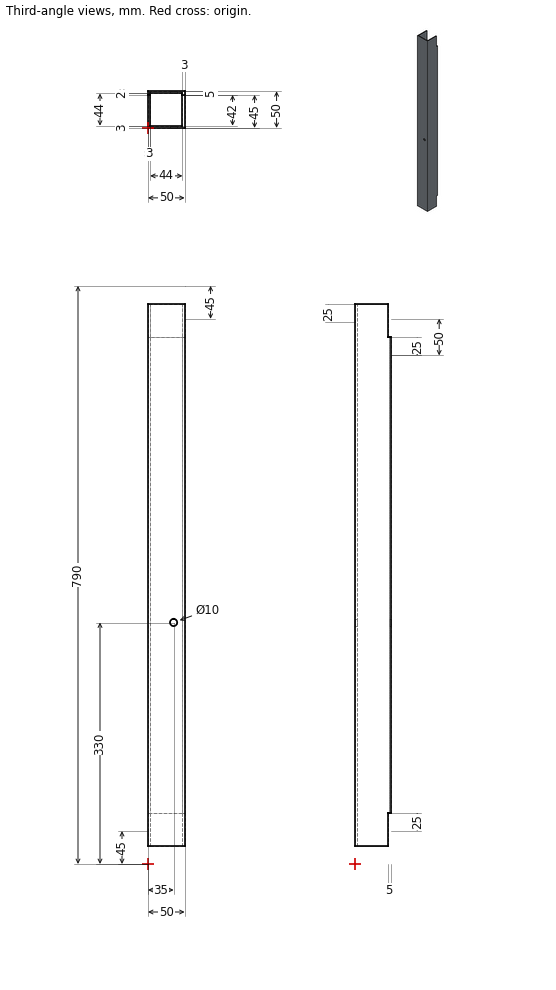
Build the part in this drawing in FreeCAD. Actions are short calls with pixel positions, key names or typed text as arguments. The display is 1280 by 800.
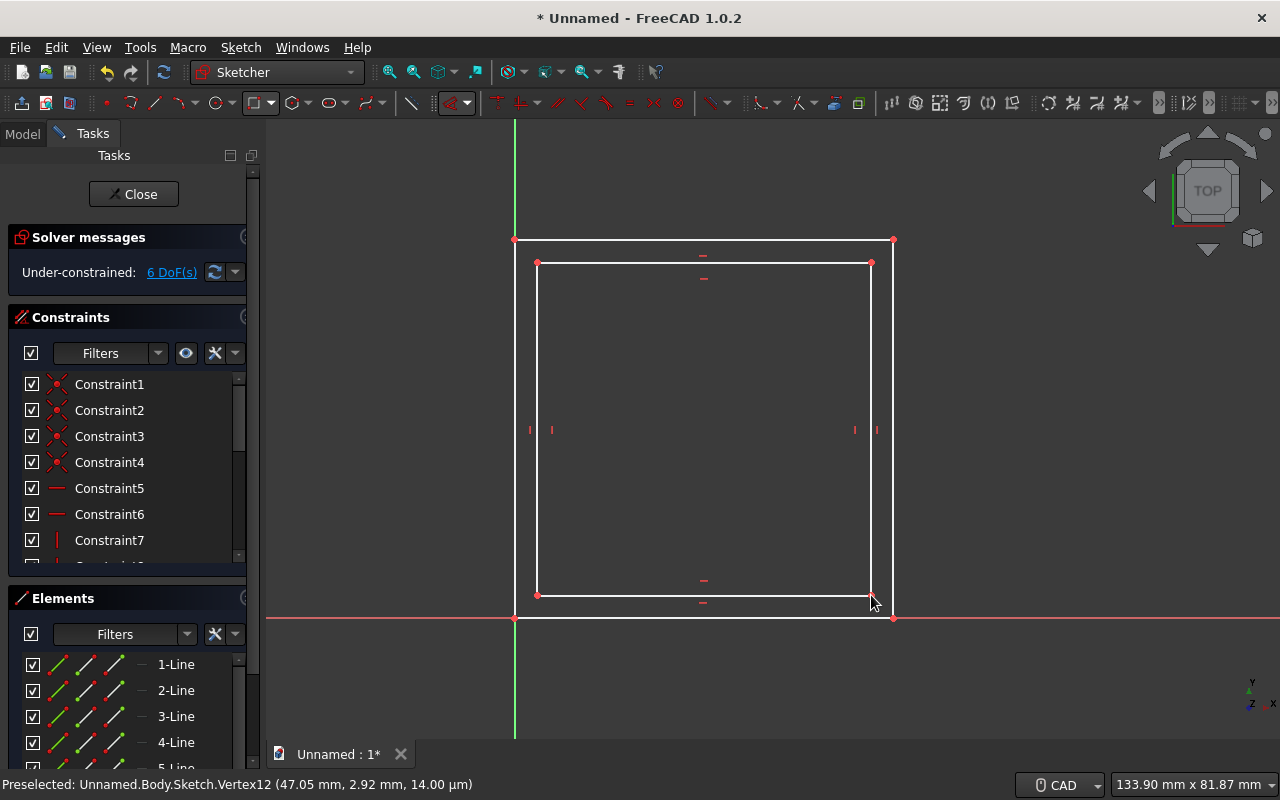
key(d)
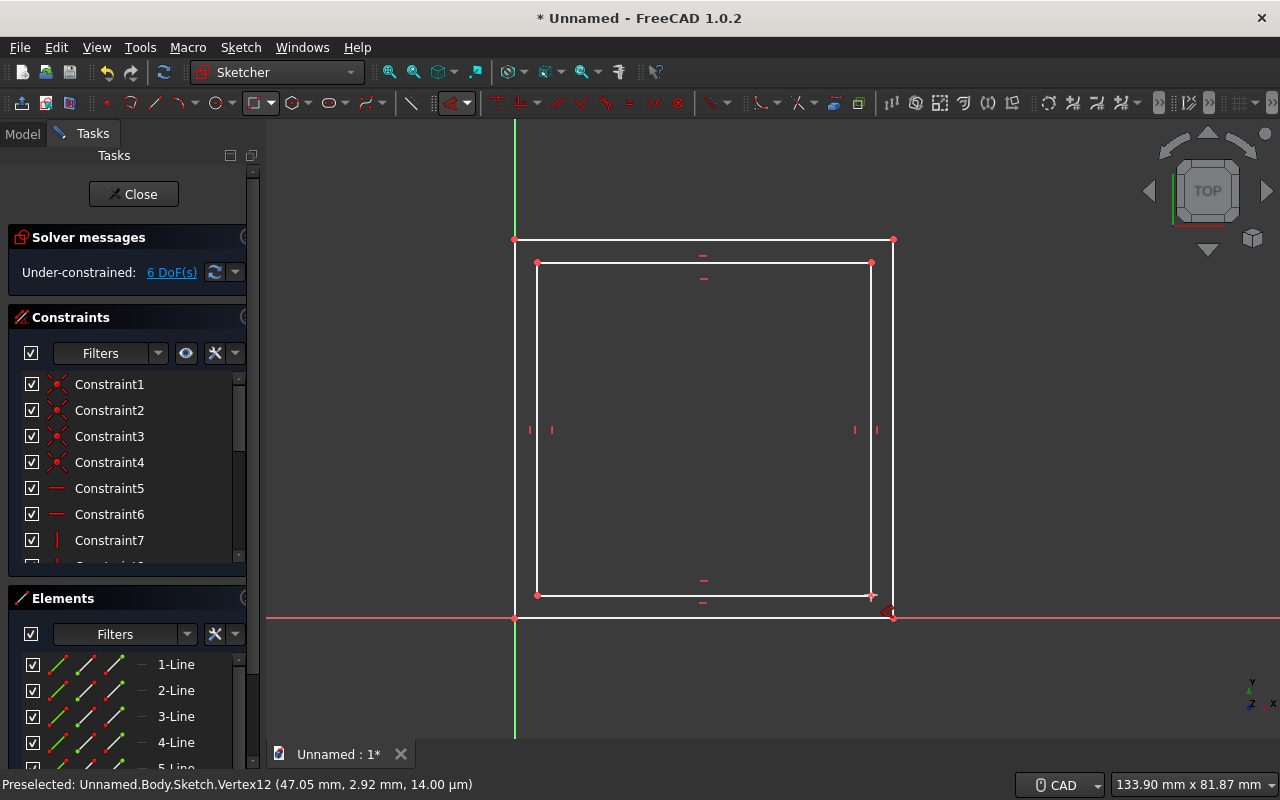
click(628, 618)
click(704, 652)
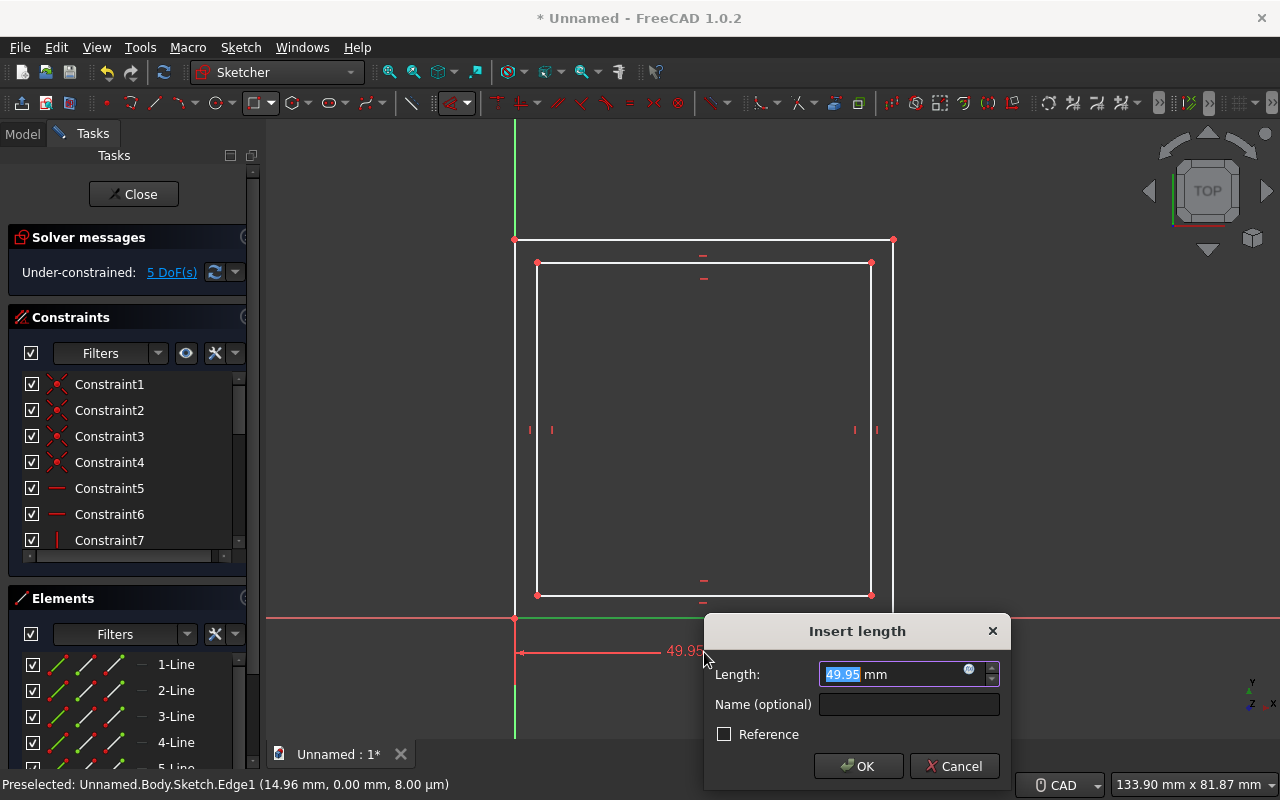
text(50)
key(Return)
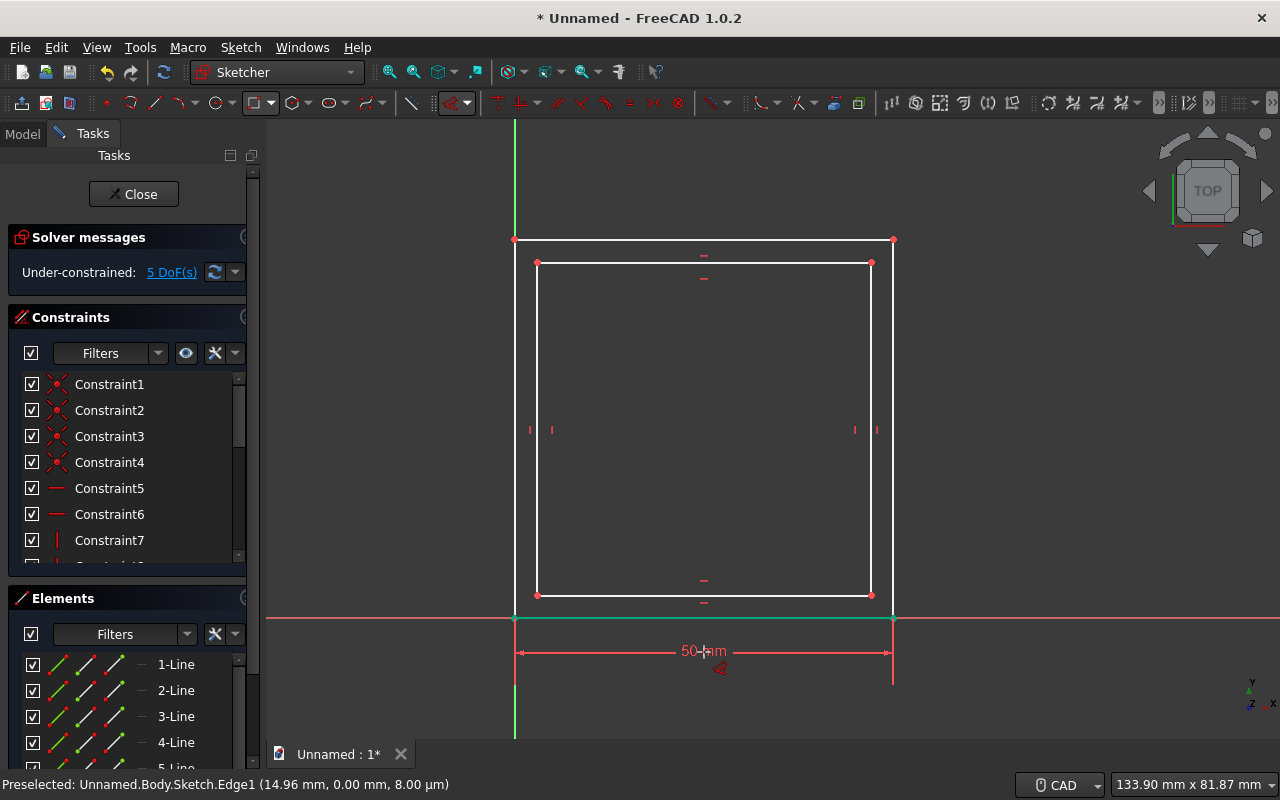
click(893, 505)
click(927, 429)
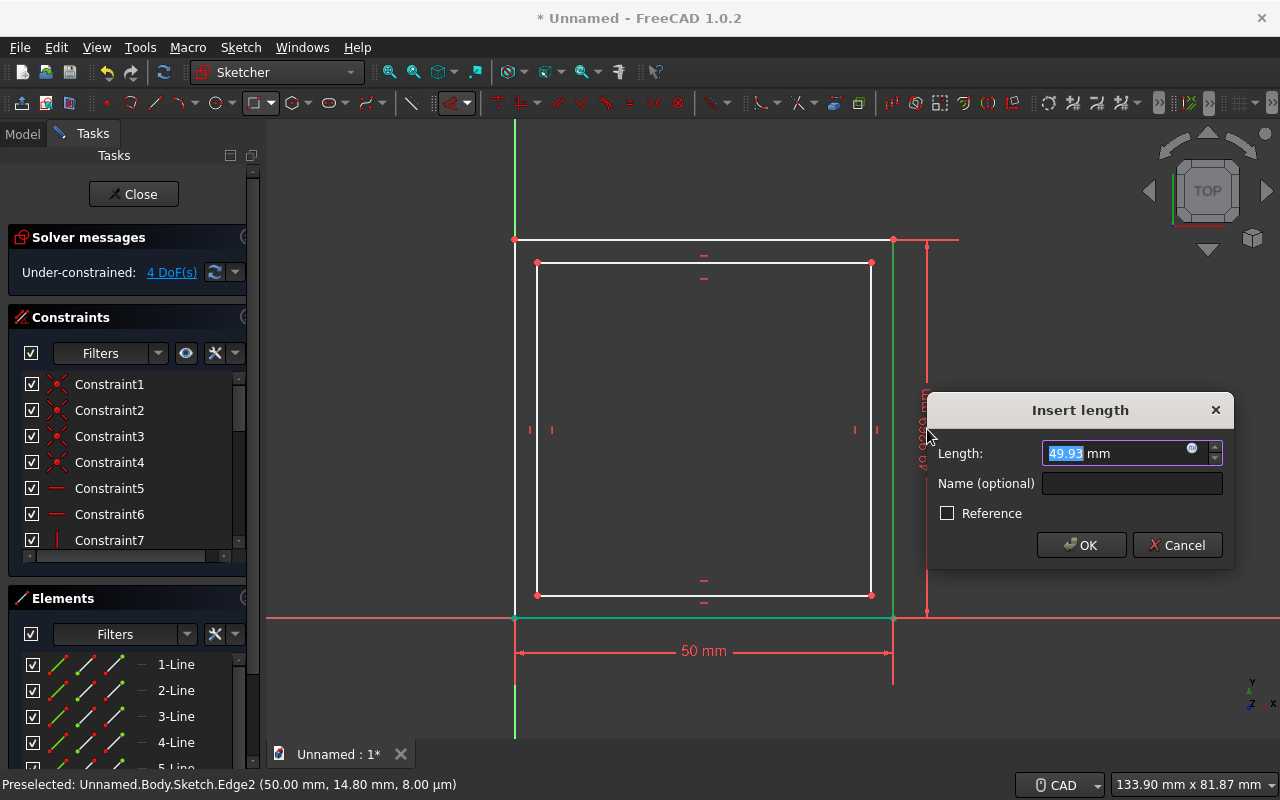
text(50)
key(Return)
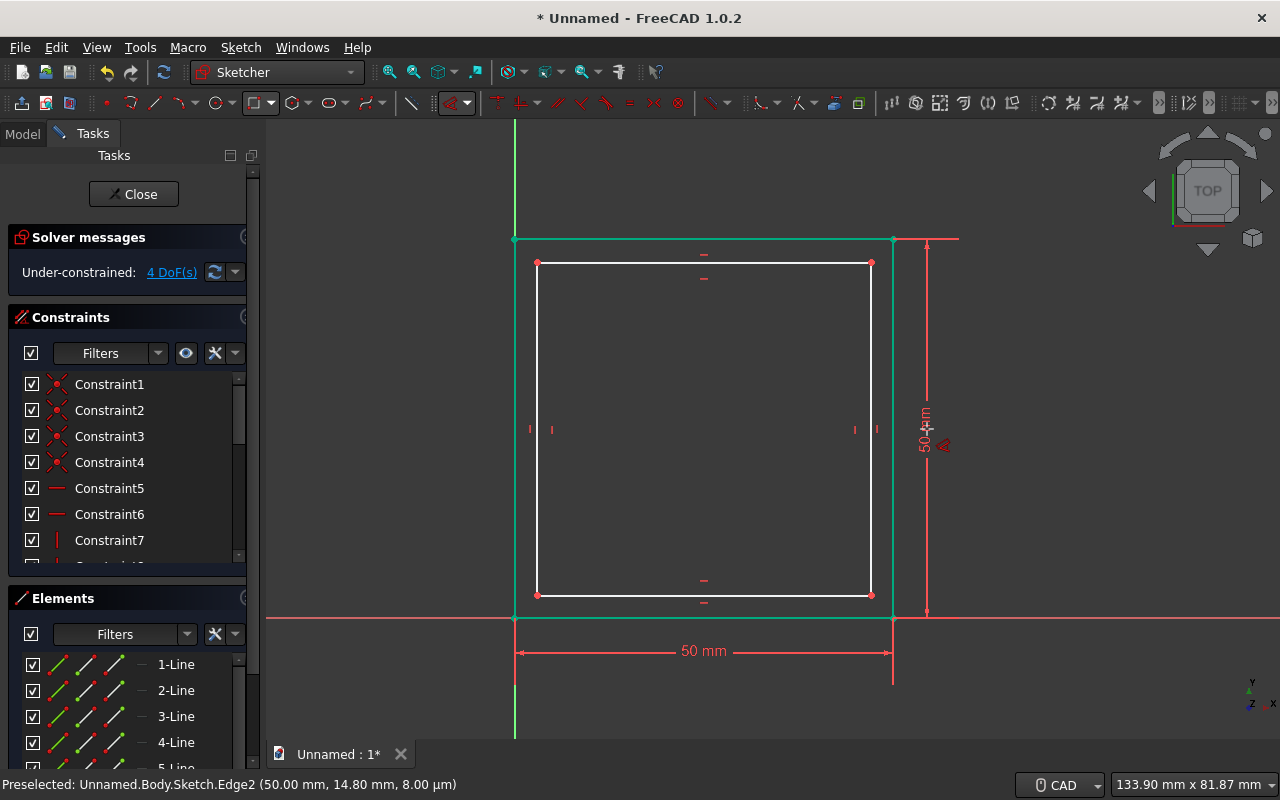
click(537, 363)
click(571, 430)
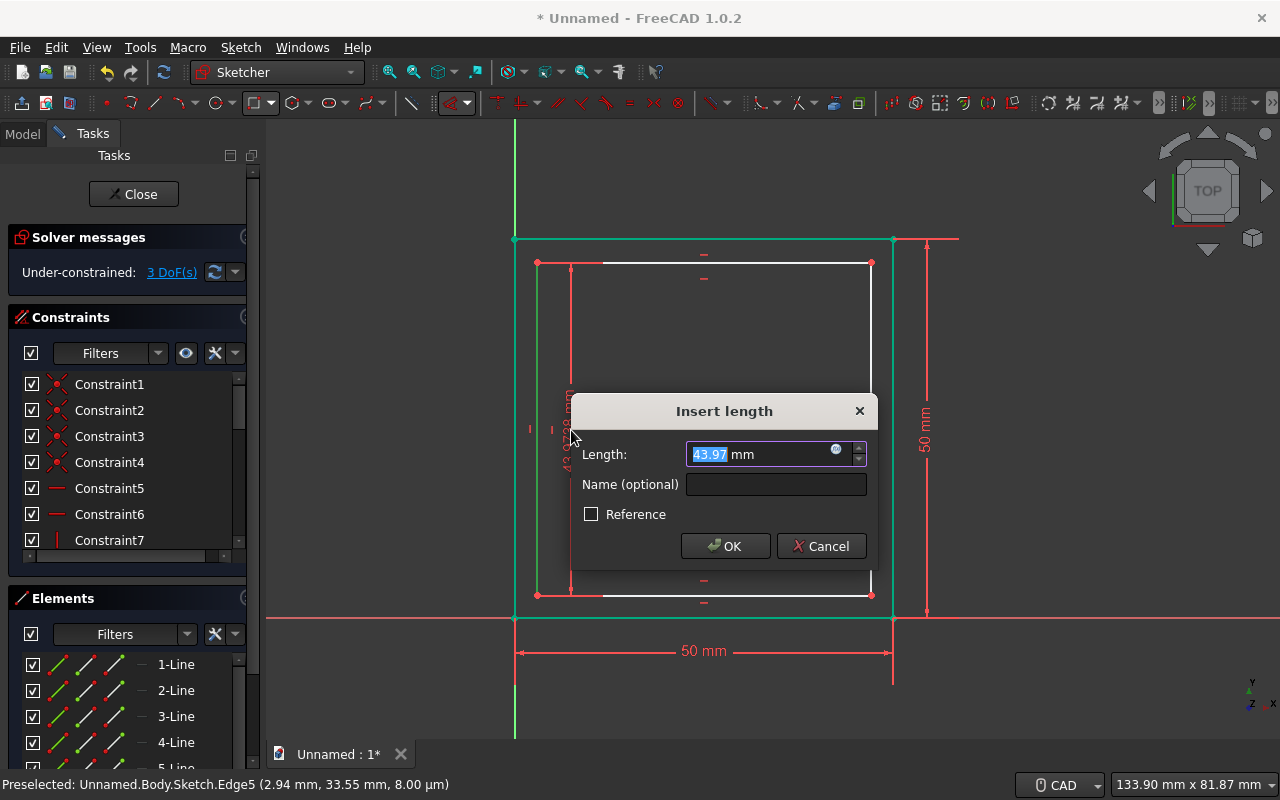
text(44)
key(Return)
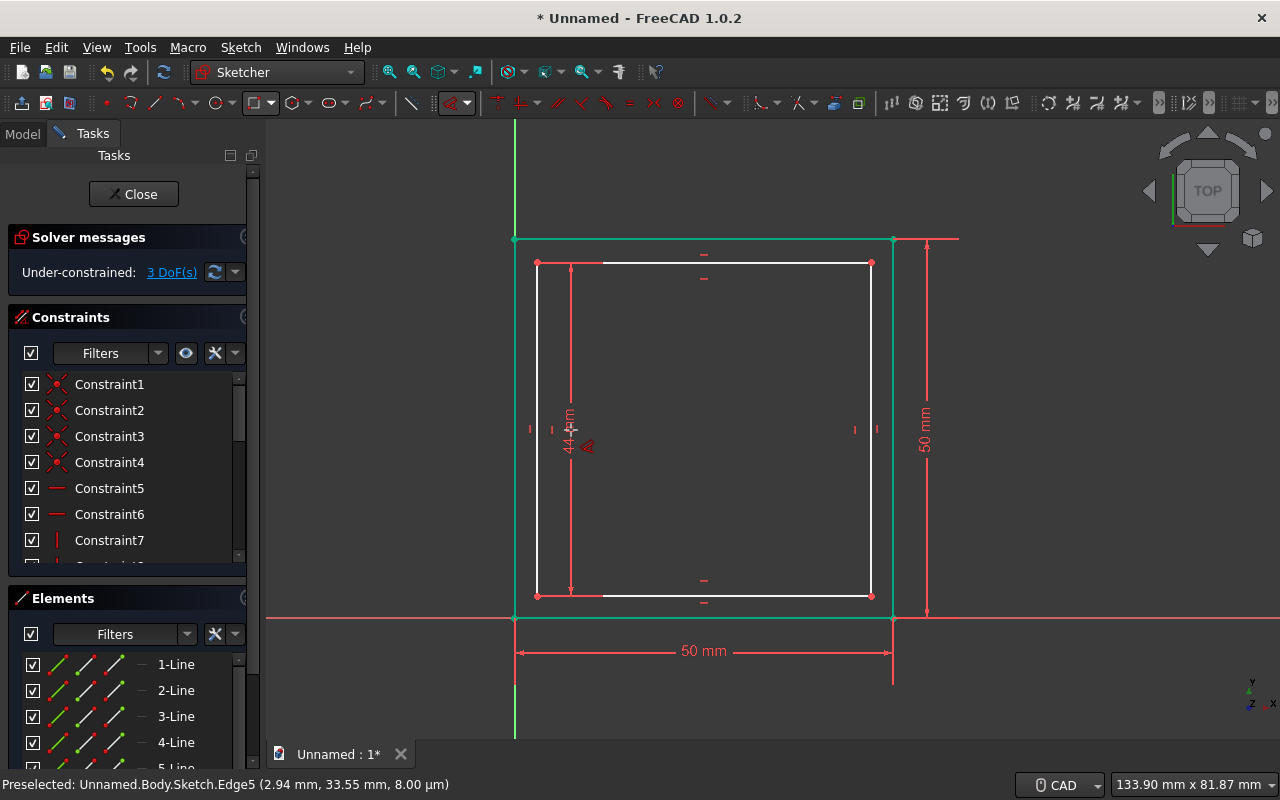
click(637, 596)
click(704, 562)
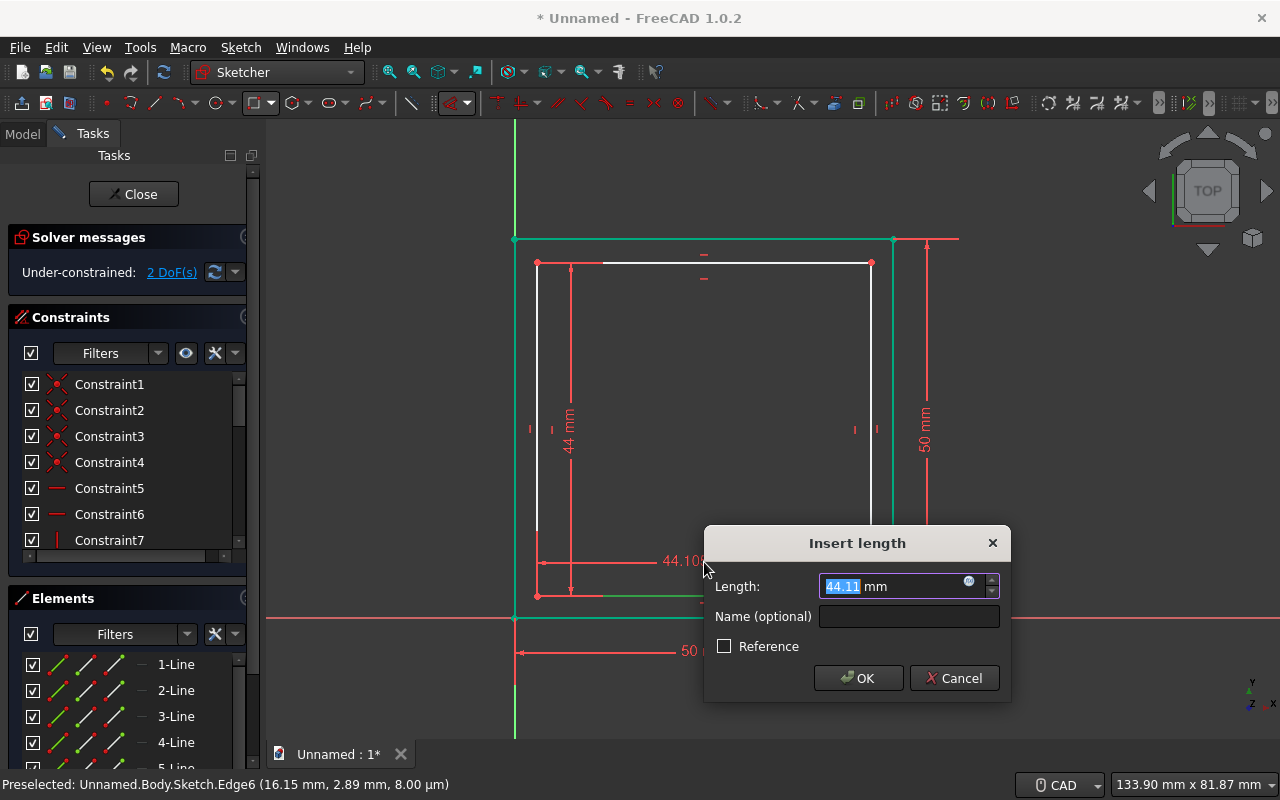
text(44)
key(Return)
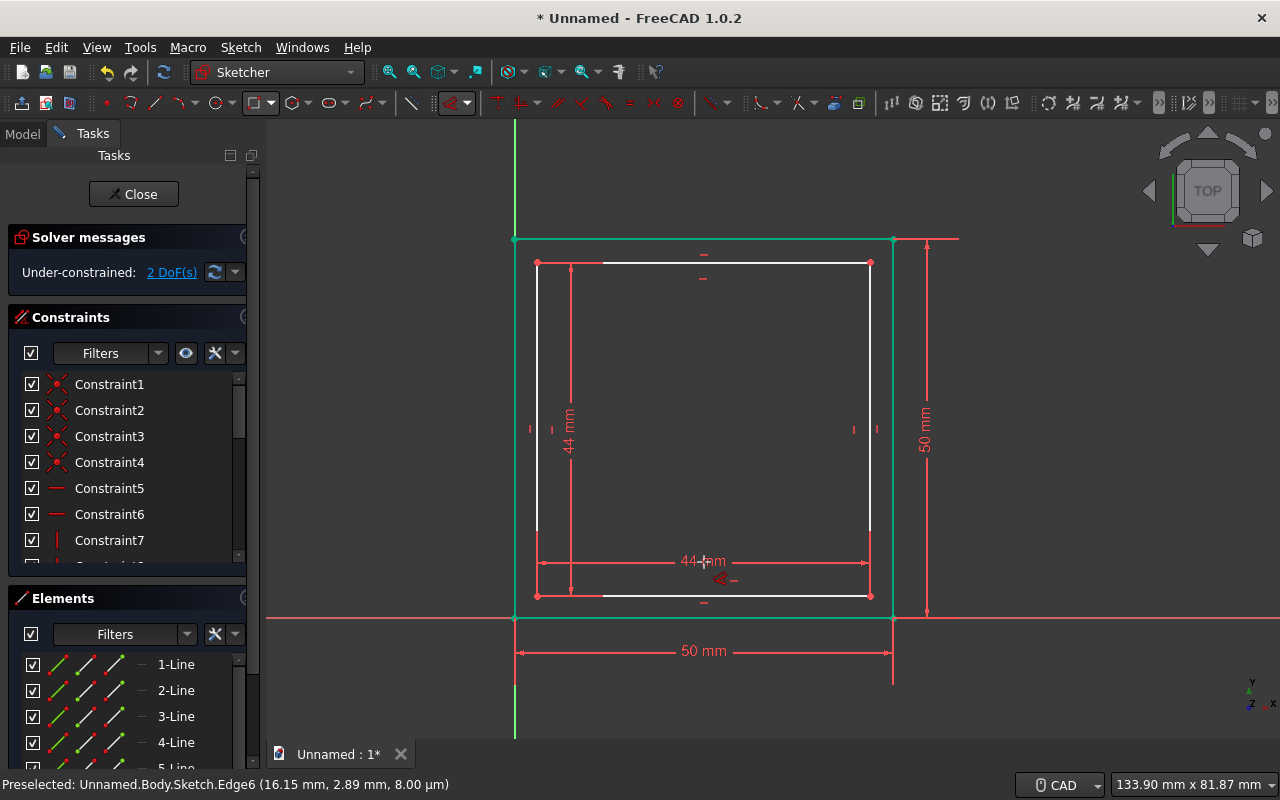
scroll(537, 263, up, 3)